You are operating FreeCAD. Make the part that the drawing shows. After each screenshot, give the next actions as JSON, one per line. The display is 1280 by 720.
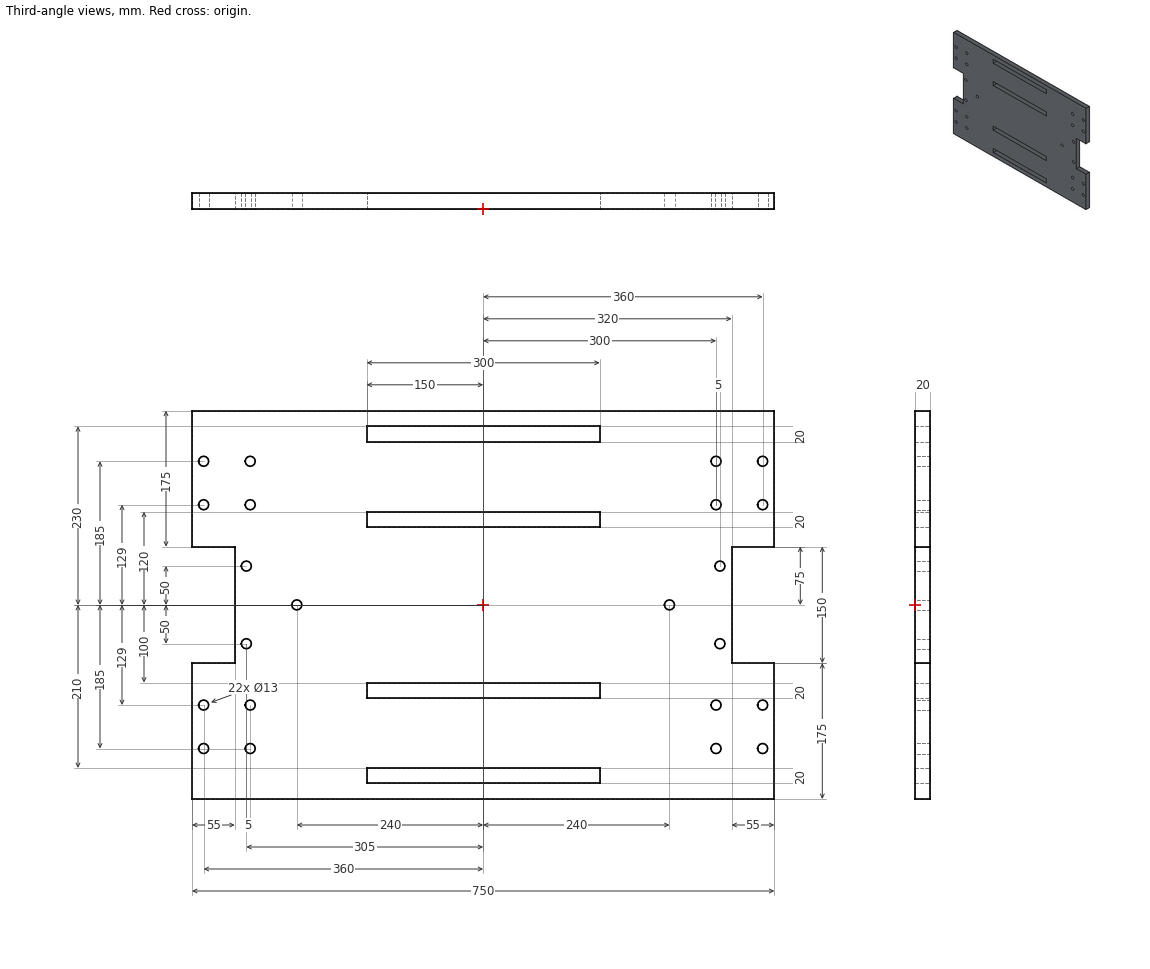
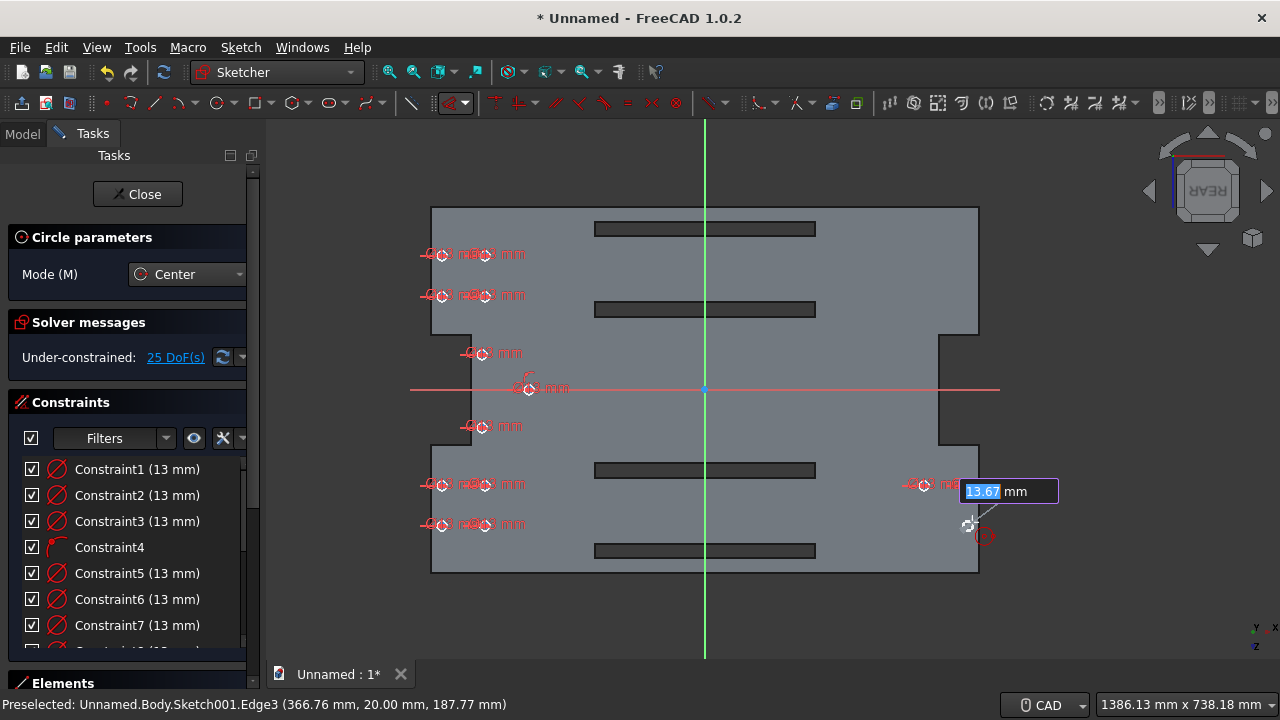
{"action": "type", "text": "13"}
{"action": "key", "text": "Return"}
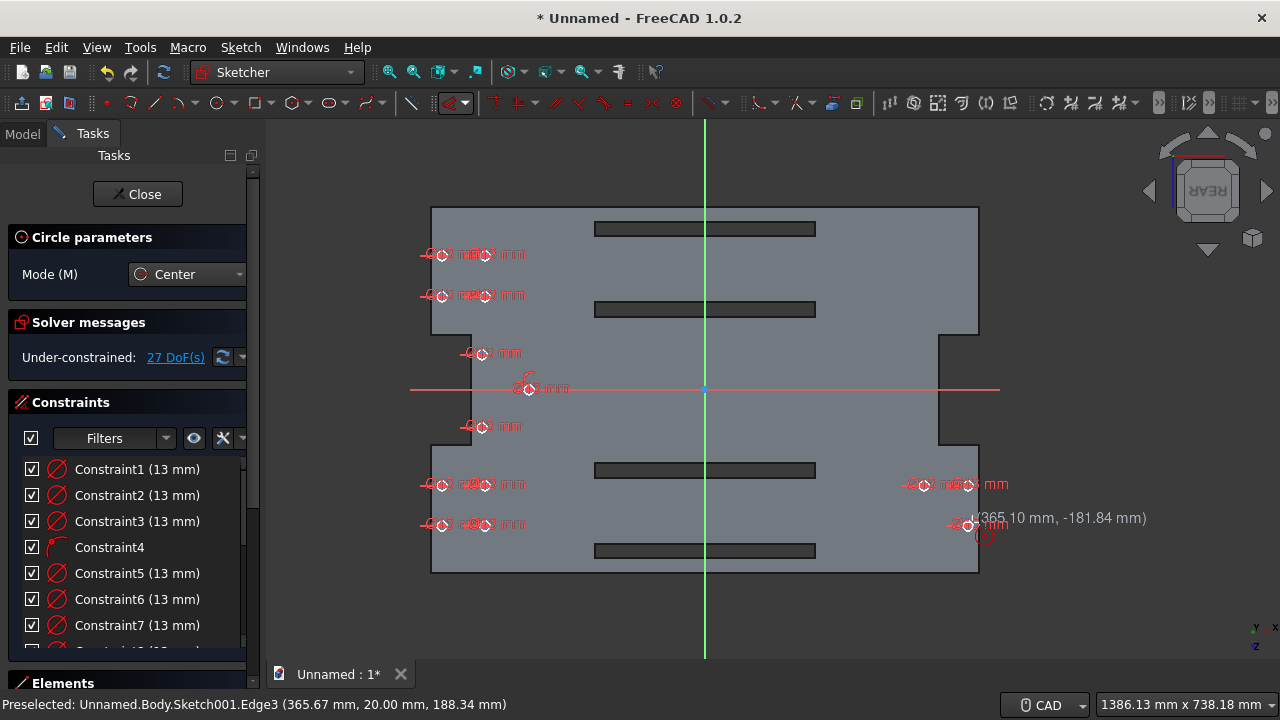
{"action": "scroll", "coordinate": [968, 296], "scroll_direction": "up", "scroll_amount": 8}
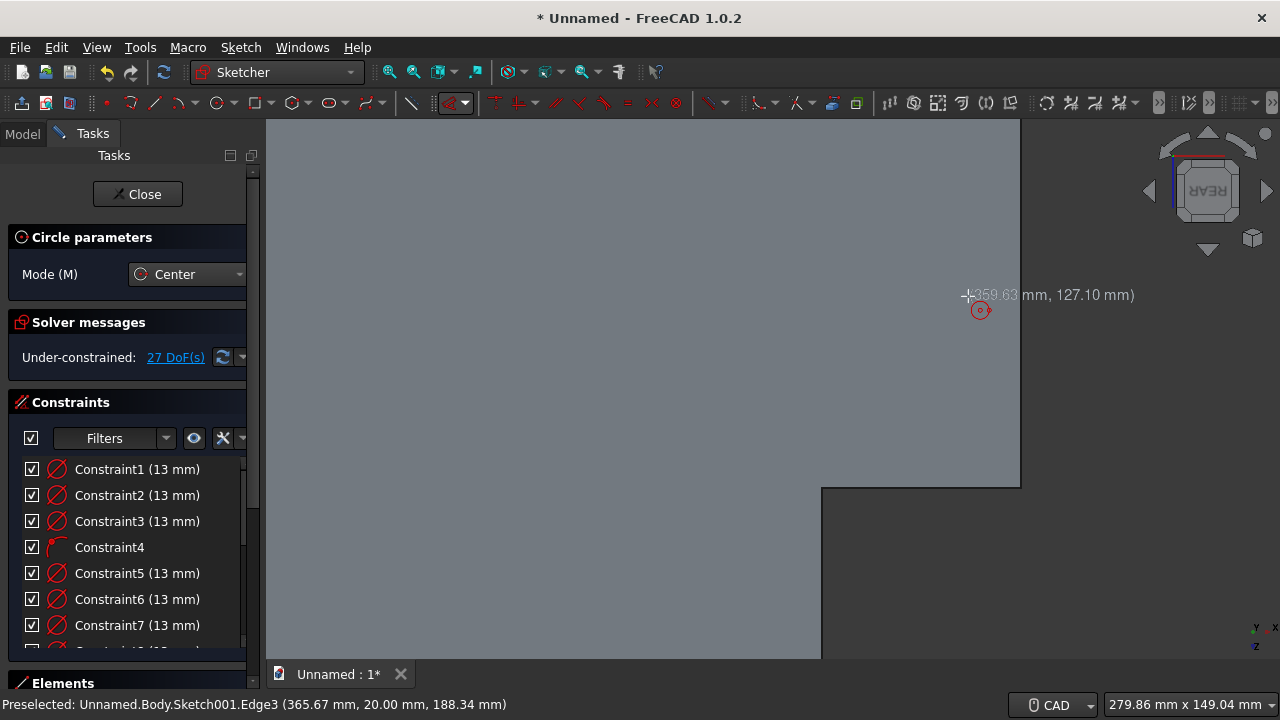
{"action": "scroll", "coordinate": [968, 295], "scroll_direction": "down", "scroll_amount": 8}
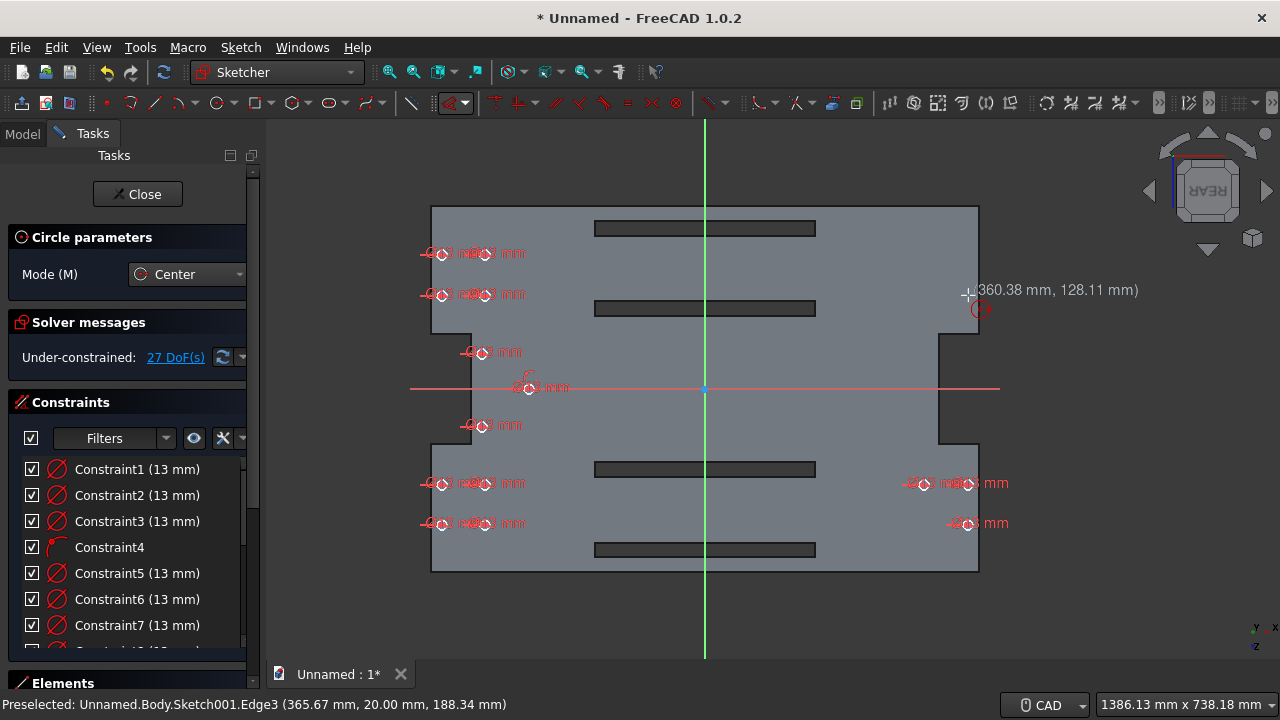
{"action": "left_click", "coordinate": [968, 295]}
{"action": "mouse_move", "coordinate": [972, 291]}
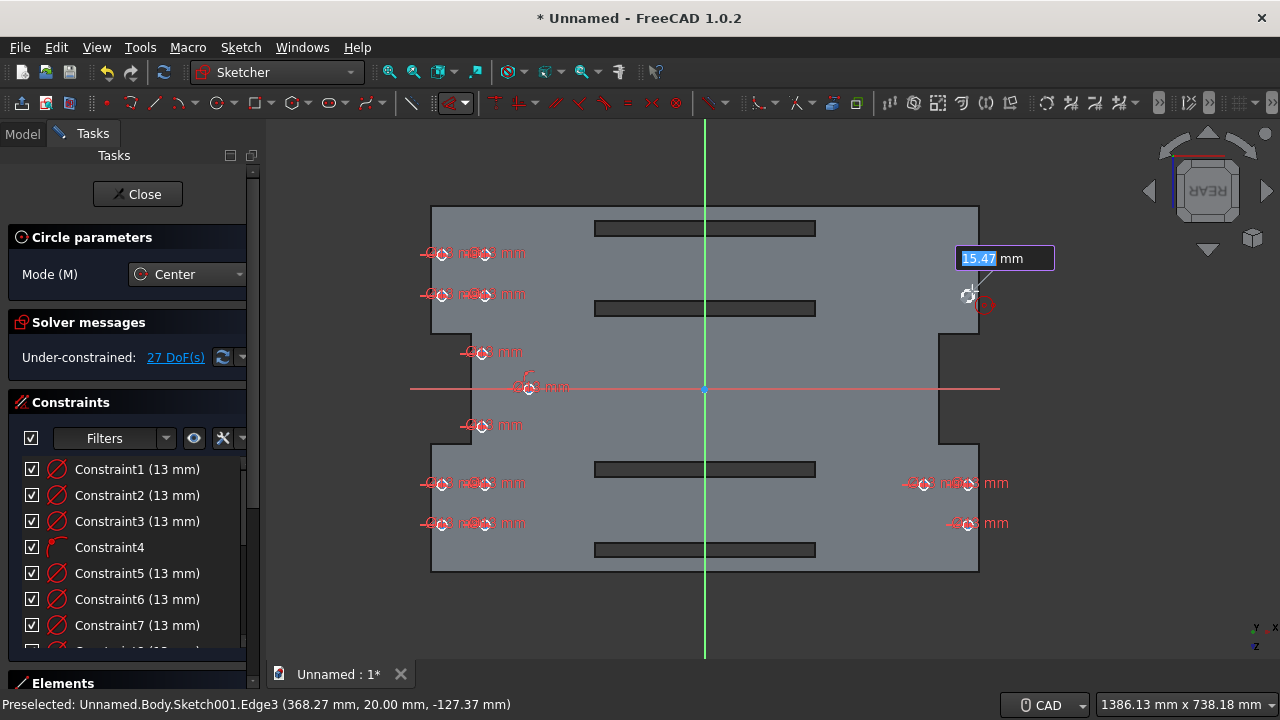
{"action": "type", "text": "13"}
{"action": "key", "text": "Return"}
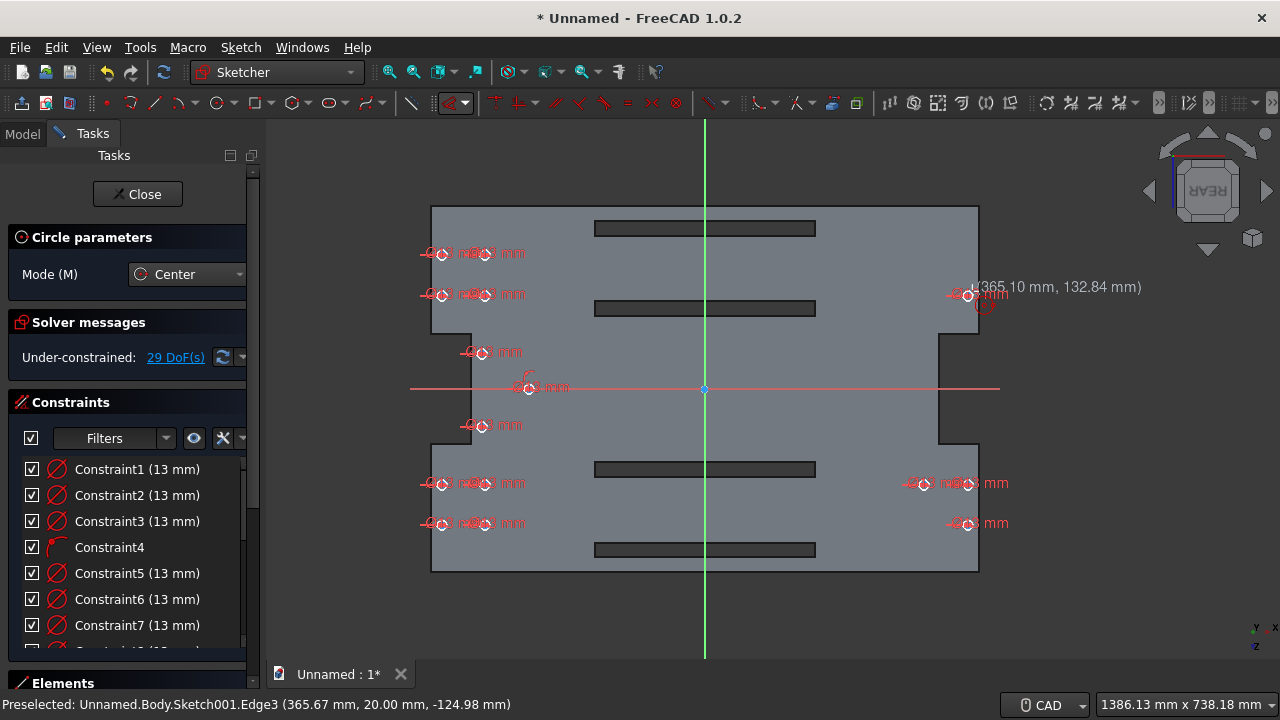
{"action": "scroll", "coordinate": [968, 254], "scroll_direction": "up", "scroll_amount": 8}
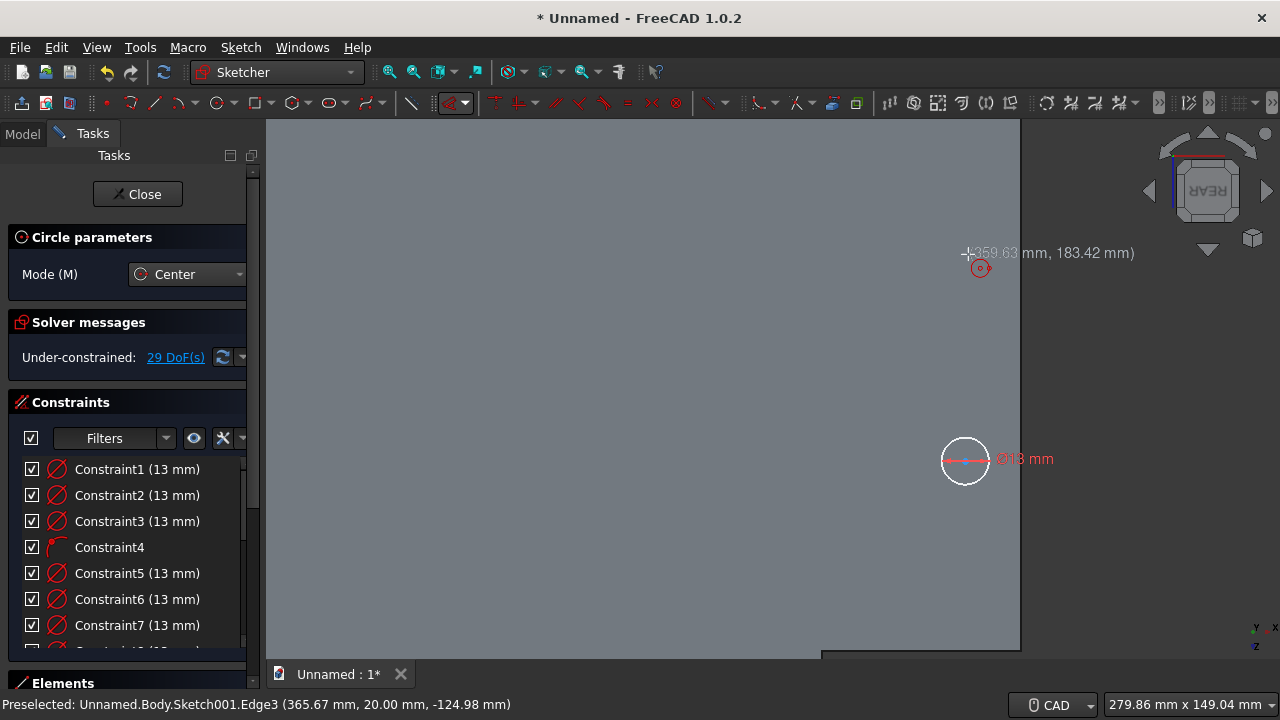
{"action": "scroll", "coordinate": [968, 254], "scroll_direction": "down", "scroll_amount": 8}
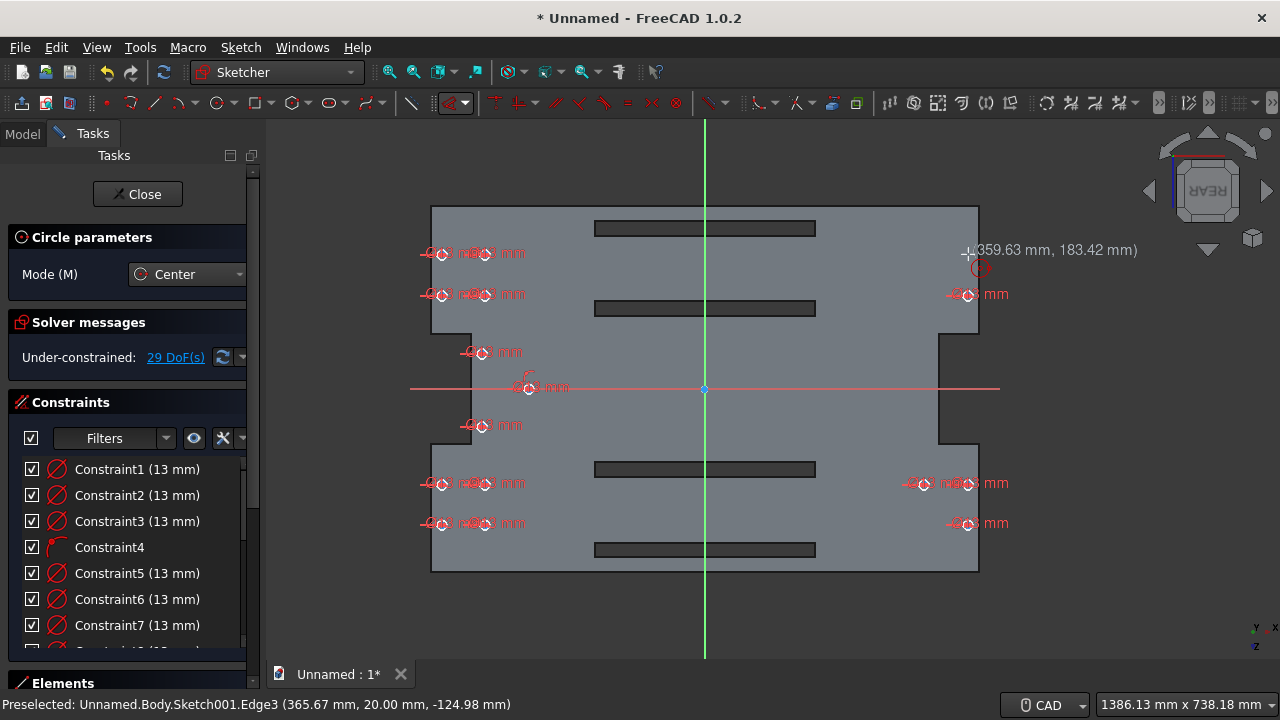
{"action": "left_click", "coordinate": [968, 254]}
{"action": "mouse_move", "coordinate": [972, 250]}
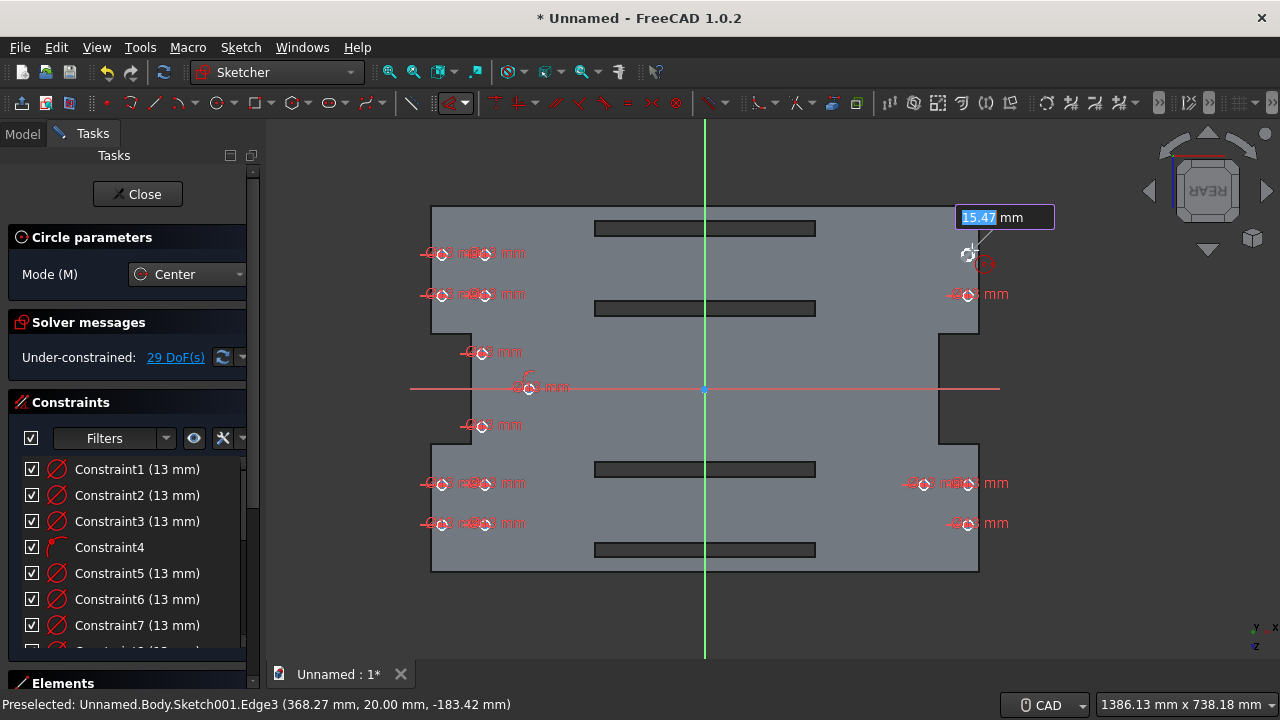
{"action": "type", "text": "13"}
{"action": "key", "text": "Return"}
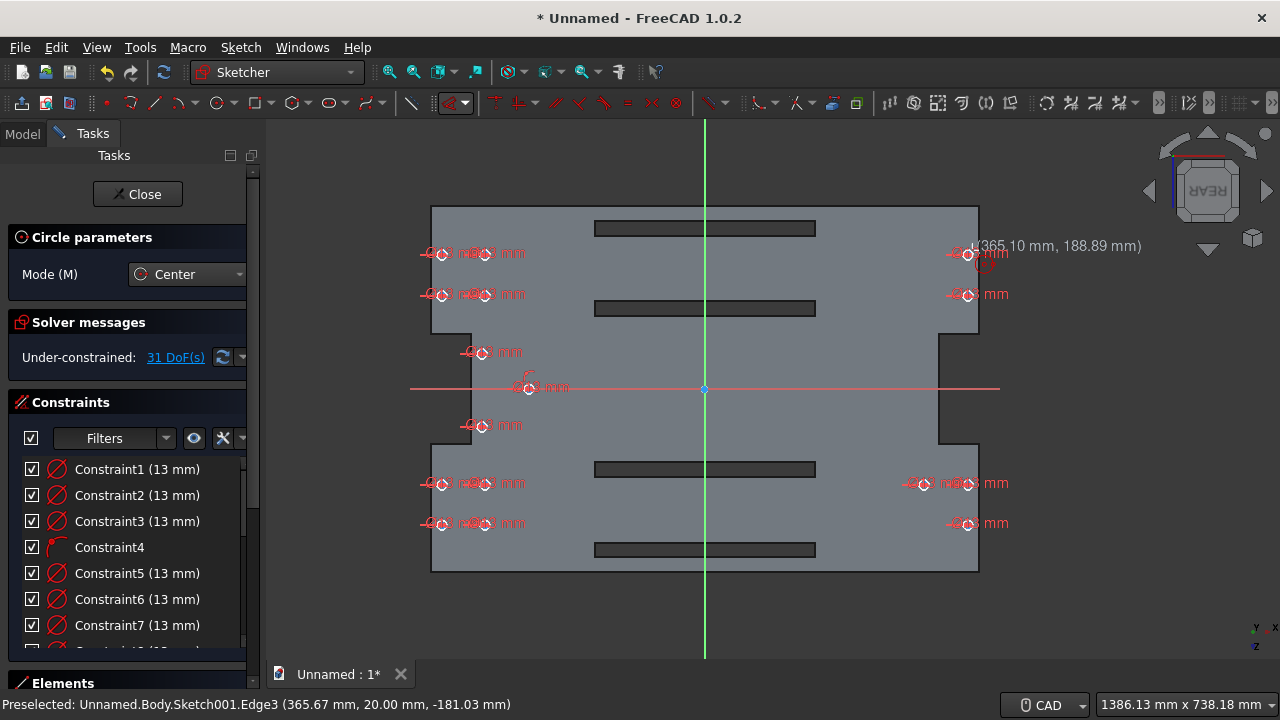
{"action": "scroll", "coordinate": [924, 295], "scroll_direction": "up", "scroll_amount": 8}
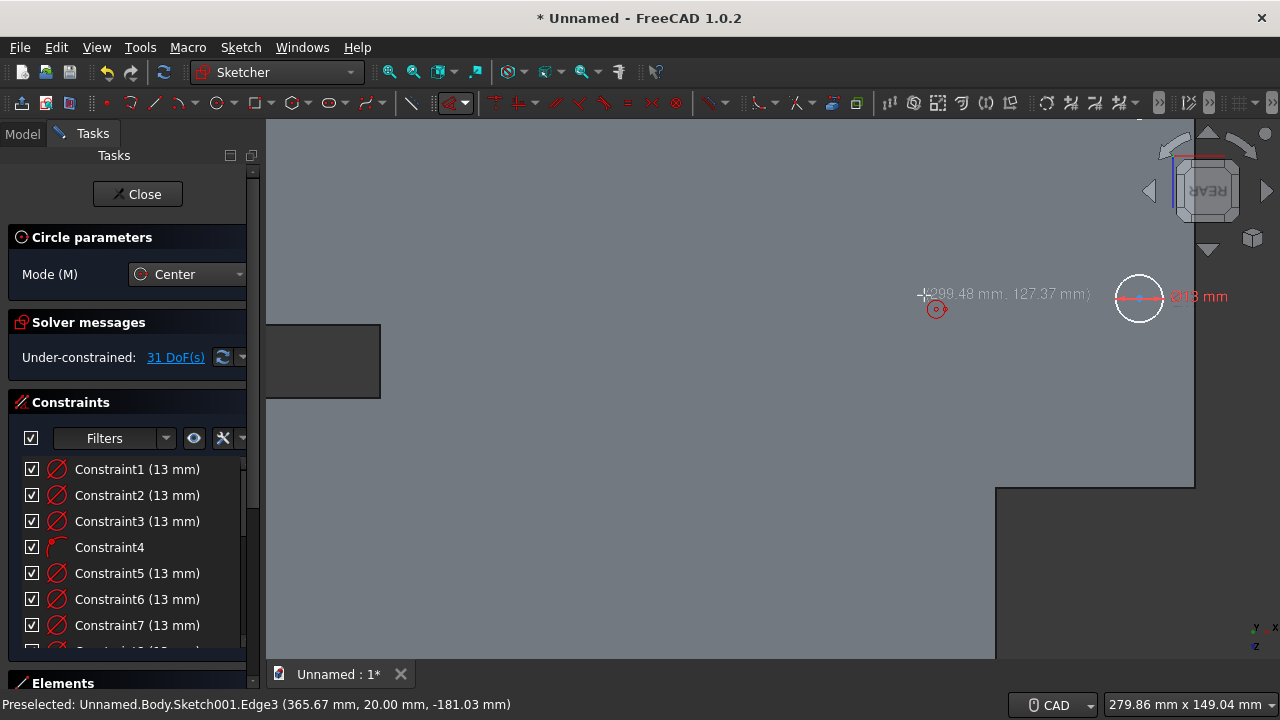
{"action": "scroll", "coordinate": [924, 295], "scroll_direction": "down", "scroll_amount": 8}